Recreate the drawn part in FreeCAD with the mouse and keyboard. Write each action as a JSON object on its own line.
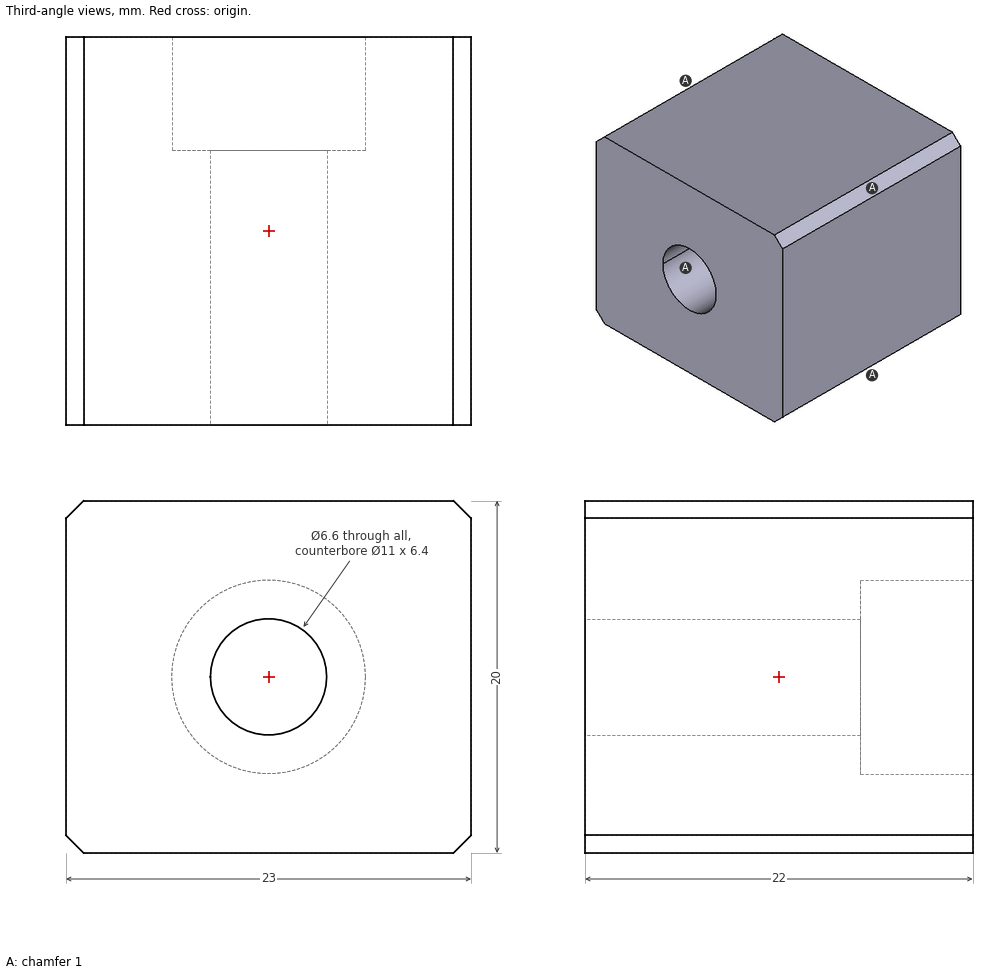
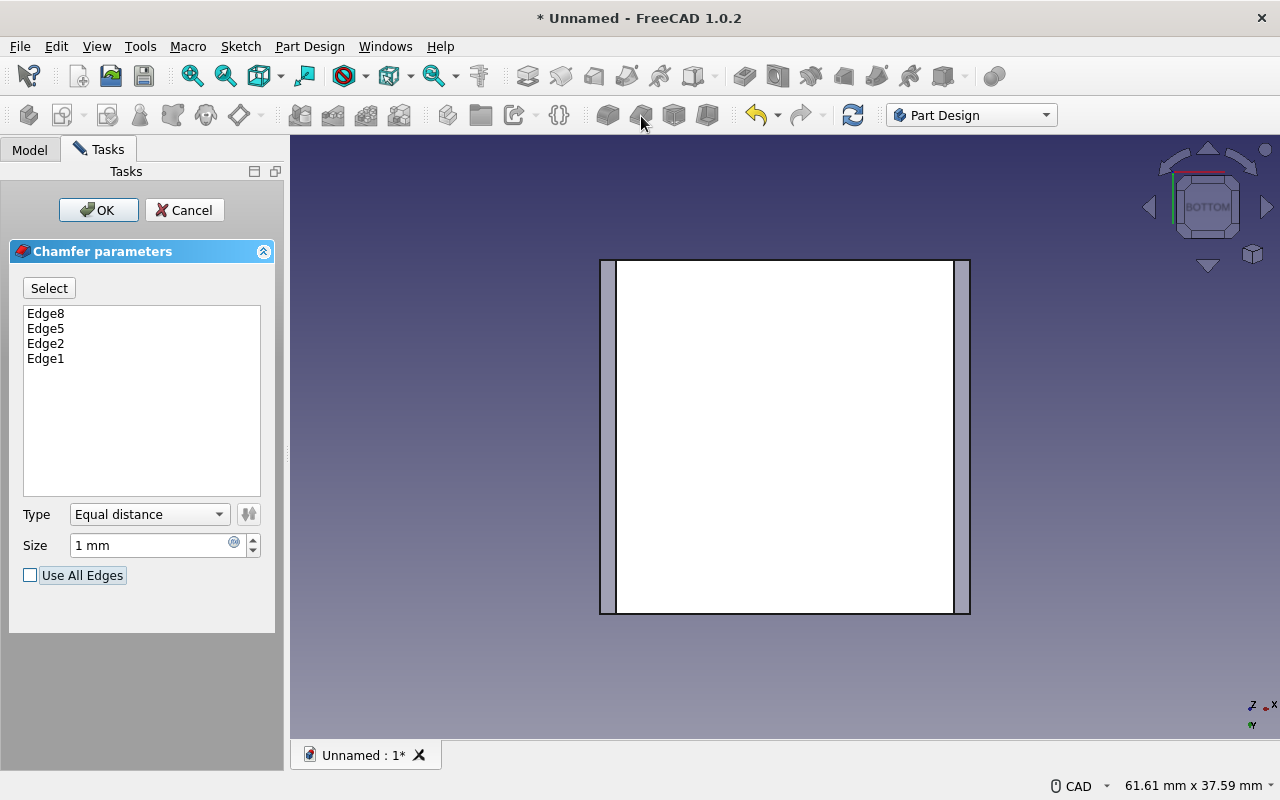
{"action": "left_click", "coordinate": [99, 210]}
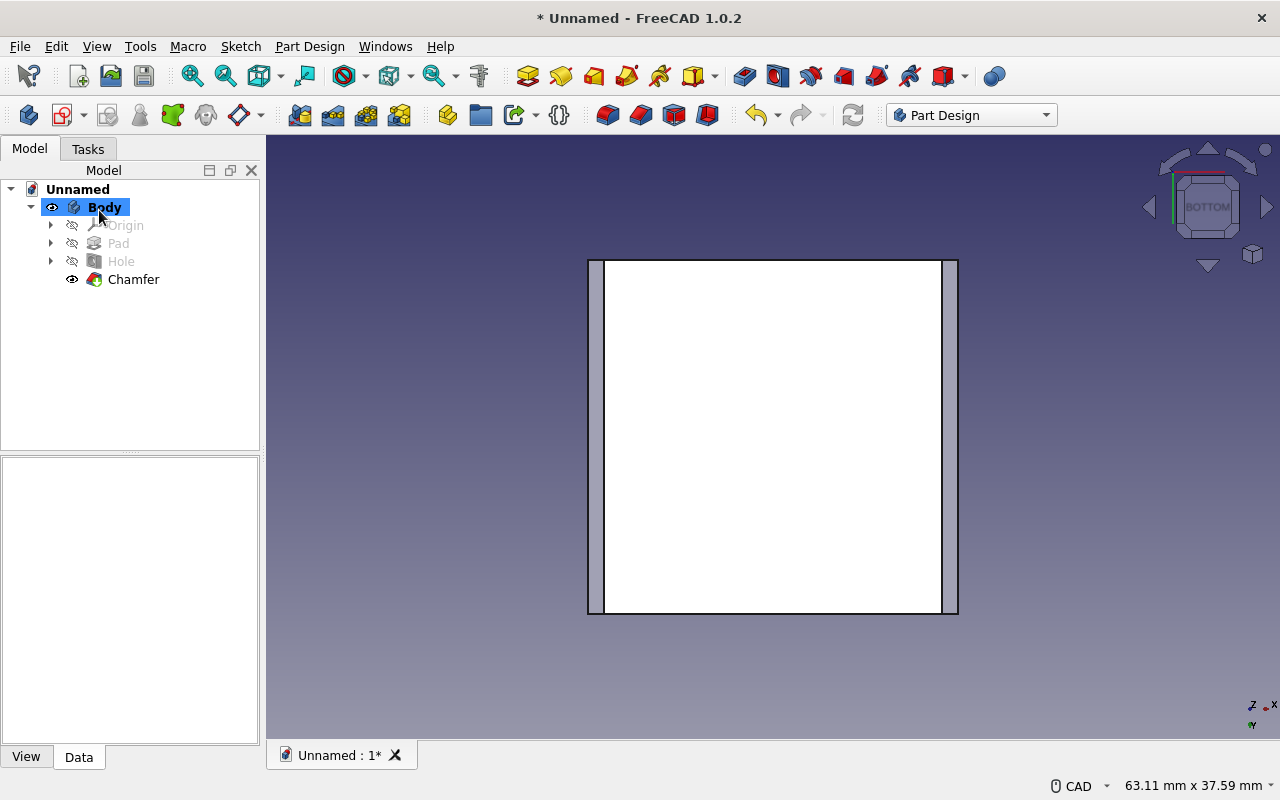
{"action": "key", "text": "0"}